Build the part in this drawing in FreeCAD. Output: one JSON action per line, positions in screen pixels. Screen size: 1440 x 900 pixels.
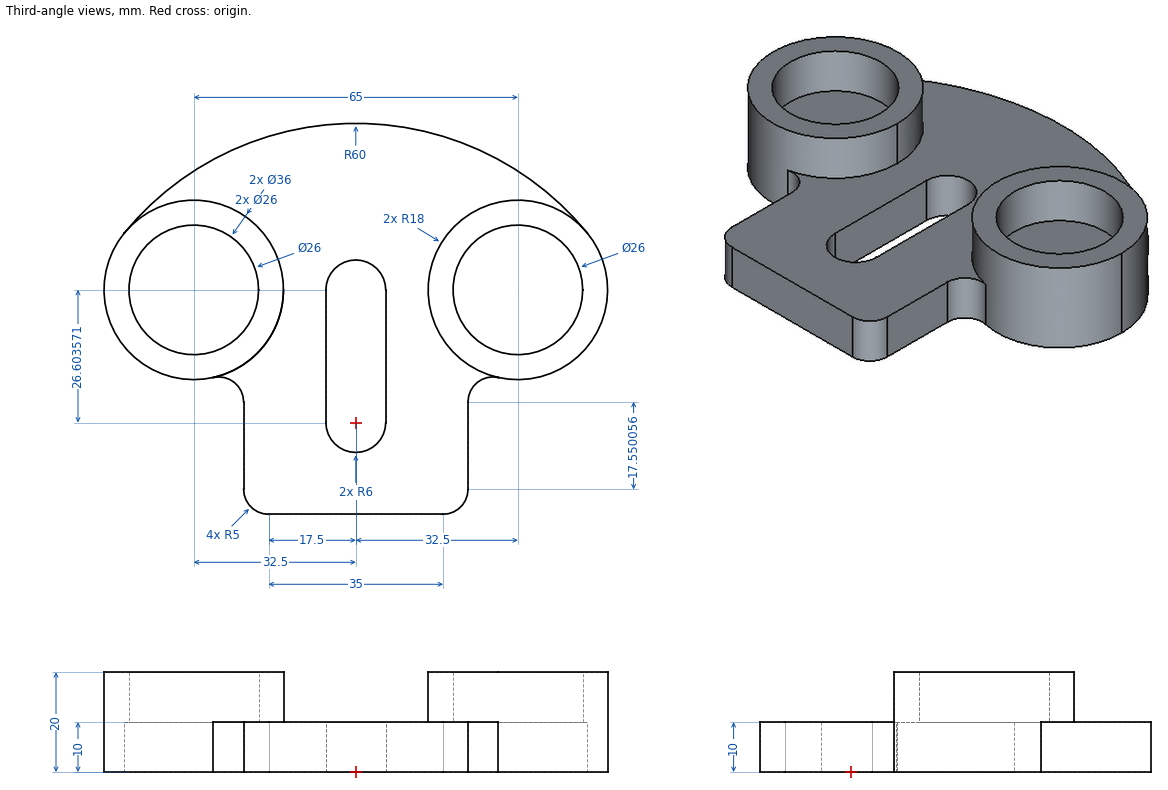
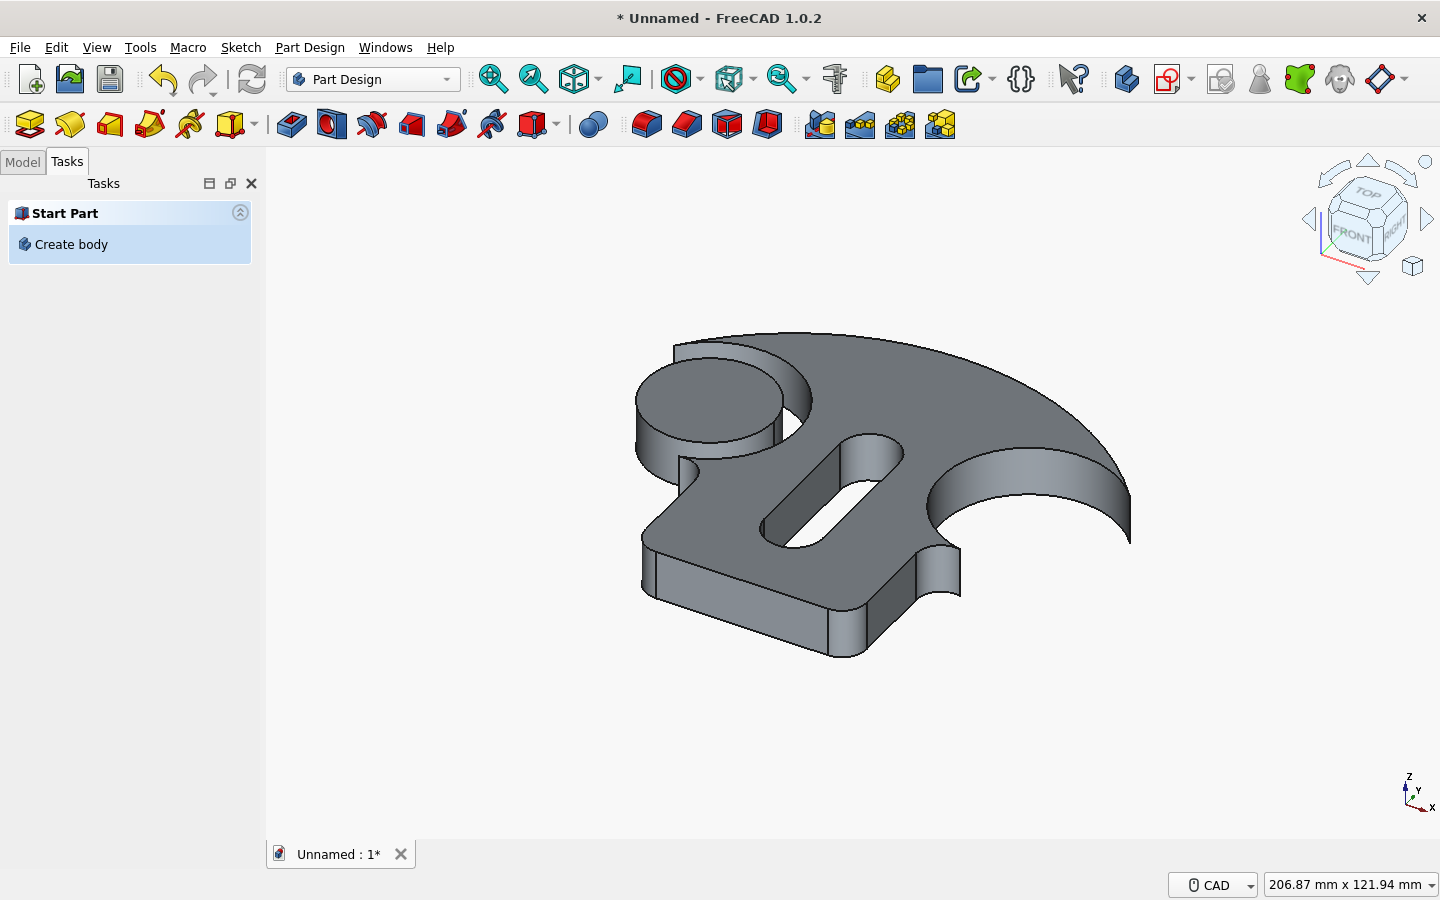
{"action": "key", "text": "v f"}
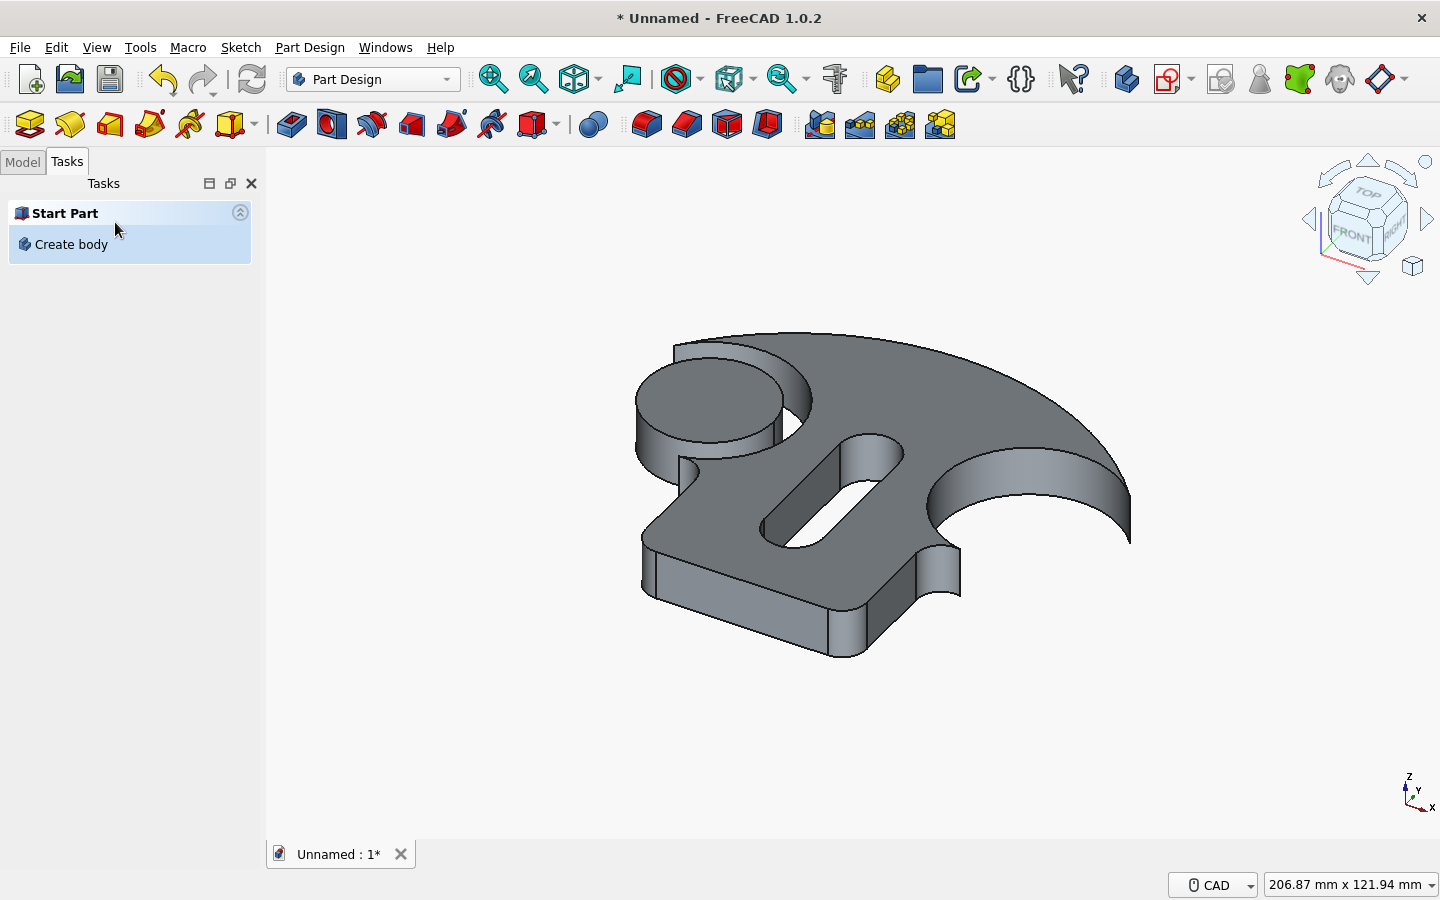
{"action": "left_click", "coordinate": [1128, 80]}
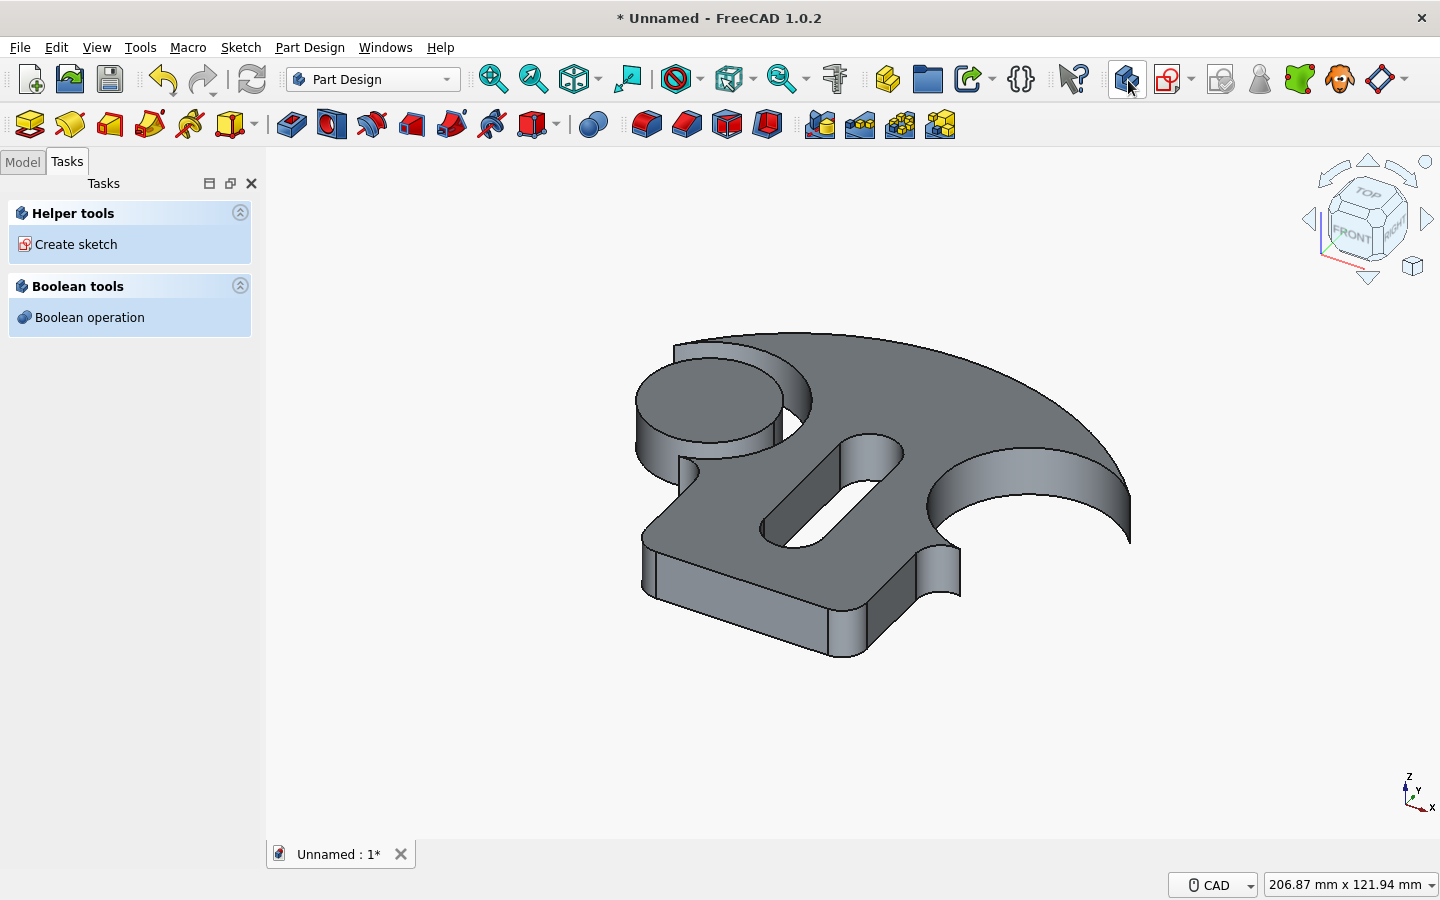
{"action": "left_click", "coordinate": [306, 799]}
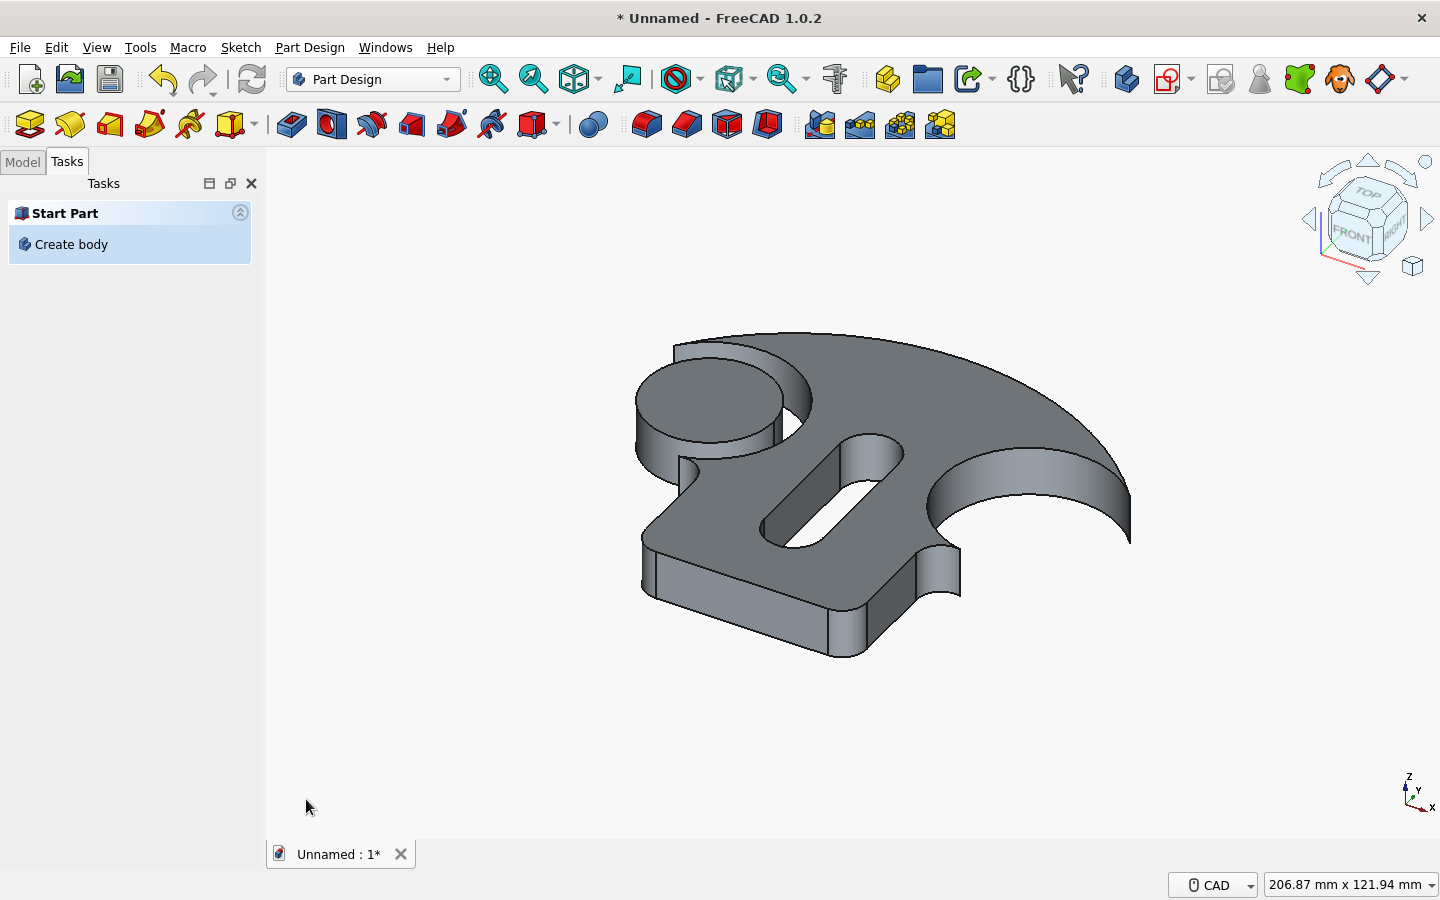
{"action": "left_click", "coordinate": [1168, 80]}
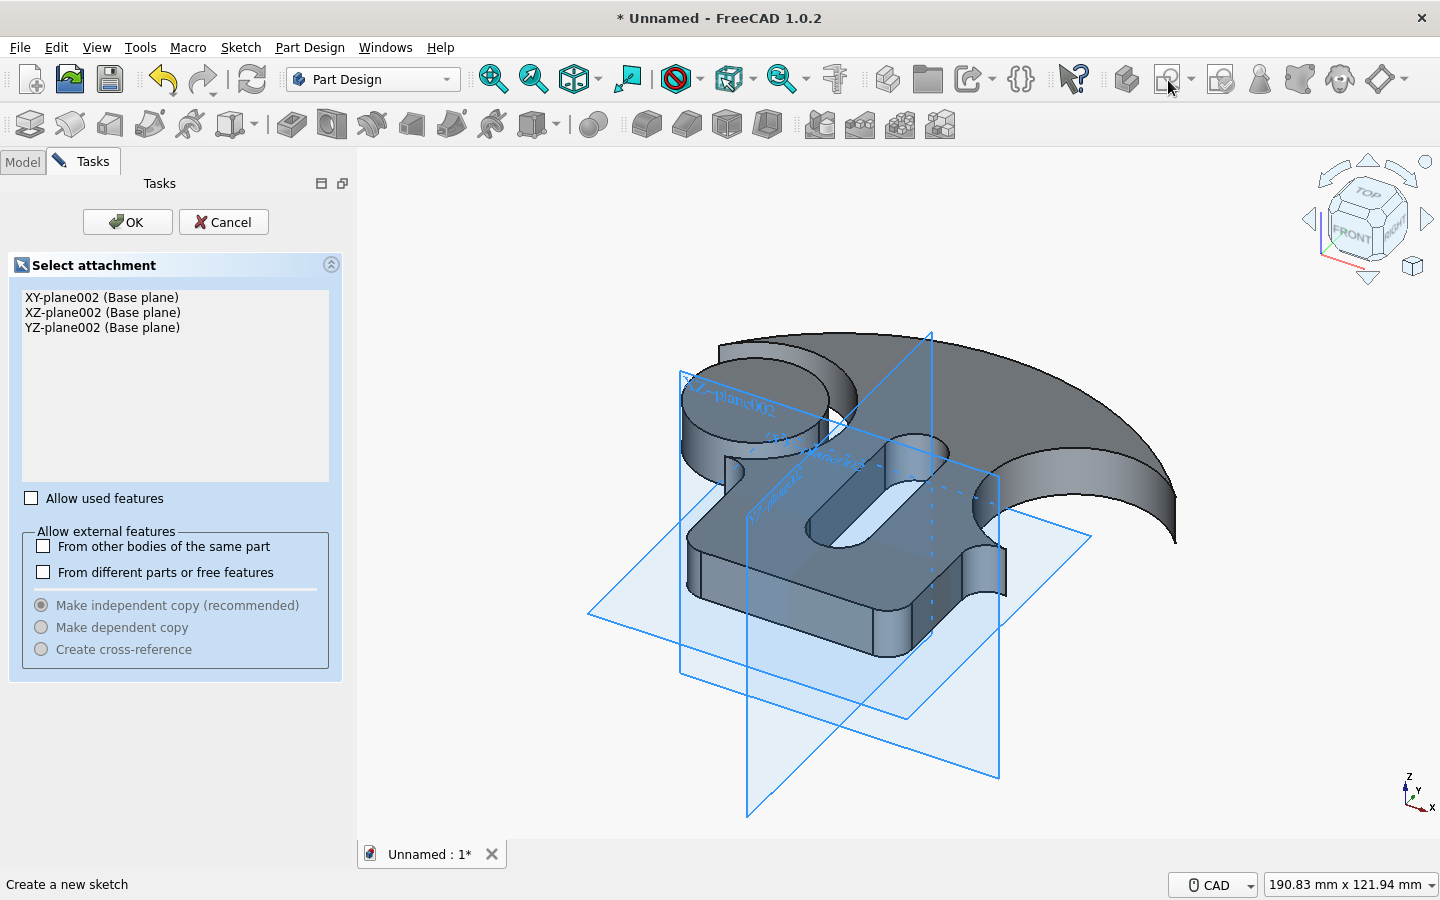
{"action": "left_click", "coordinate": [82, 298]}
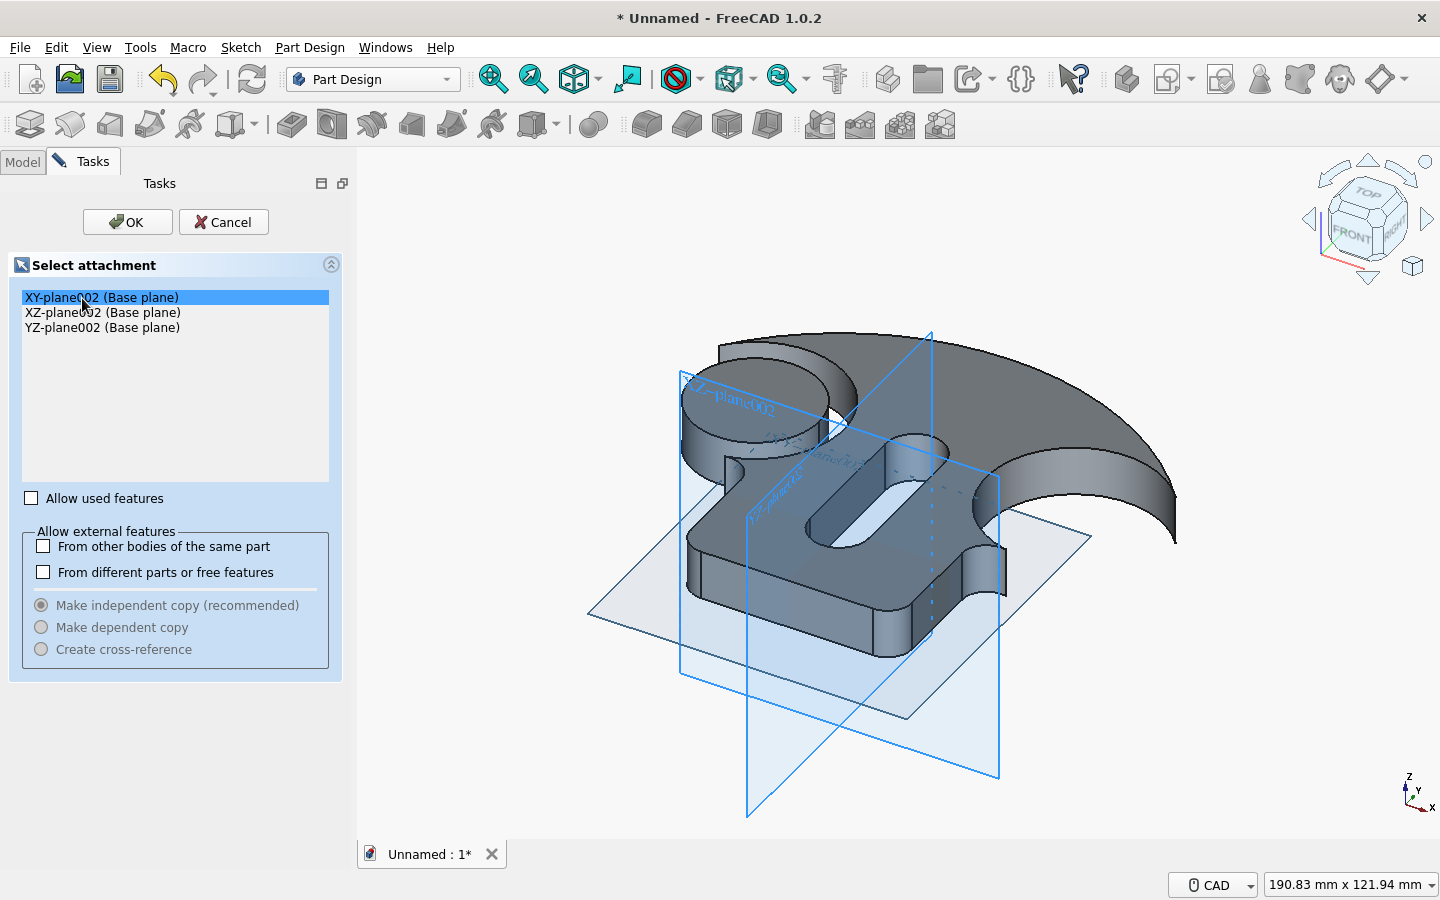
{"action": "left_click", "coordinate": [128, 222]}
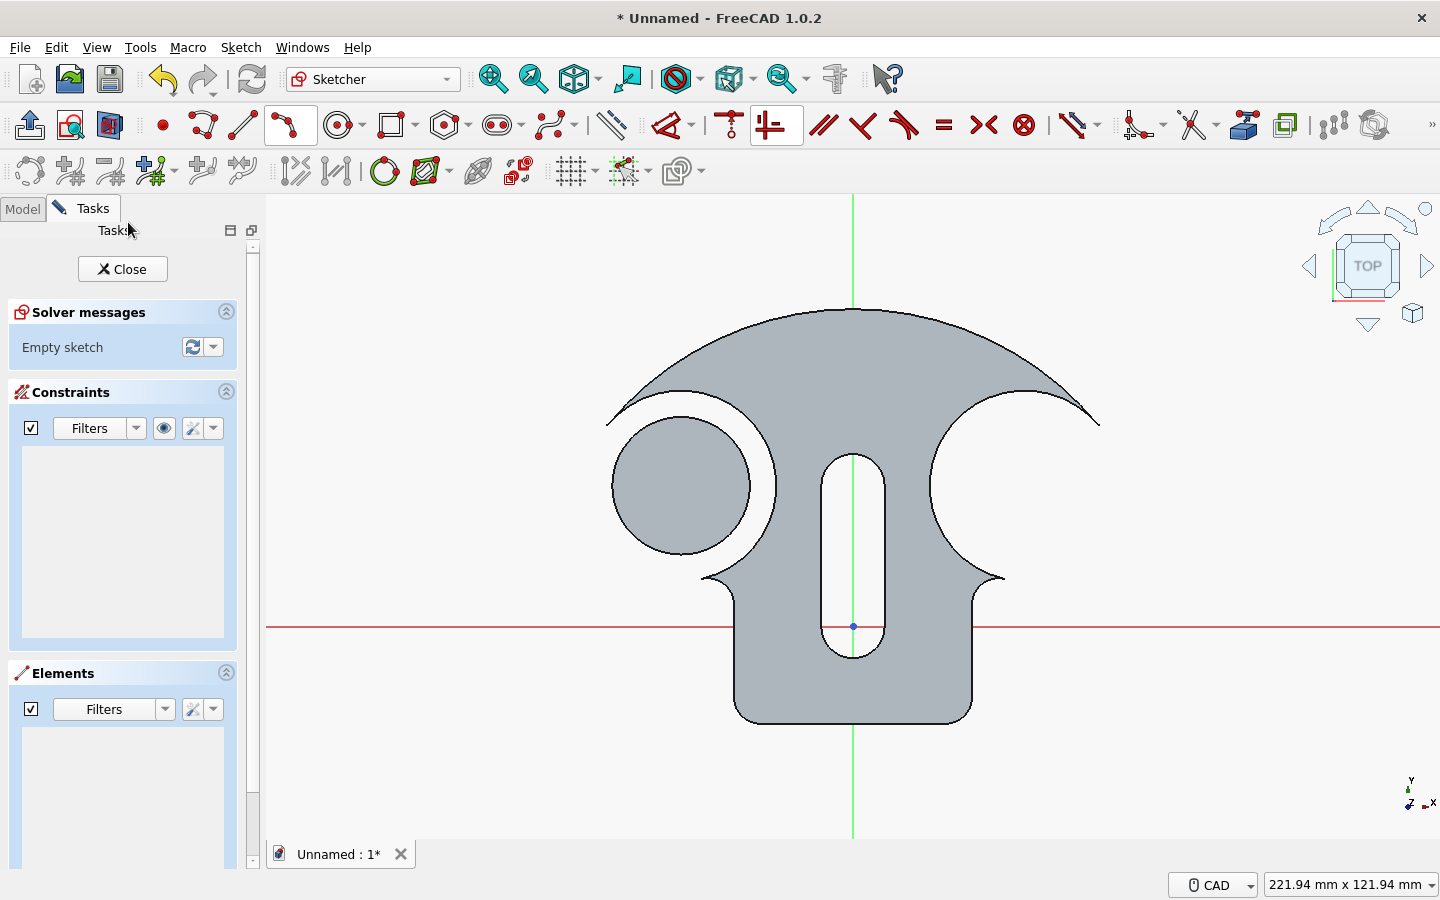
{"action": "scroll", "coordinate": [1203, 528], "scroll_direction": "up", "scroll_amount": 3}